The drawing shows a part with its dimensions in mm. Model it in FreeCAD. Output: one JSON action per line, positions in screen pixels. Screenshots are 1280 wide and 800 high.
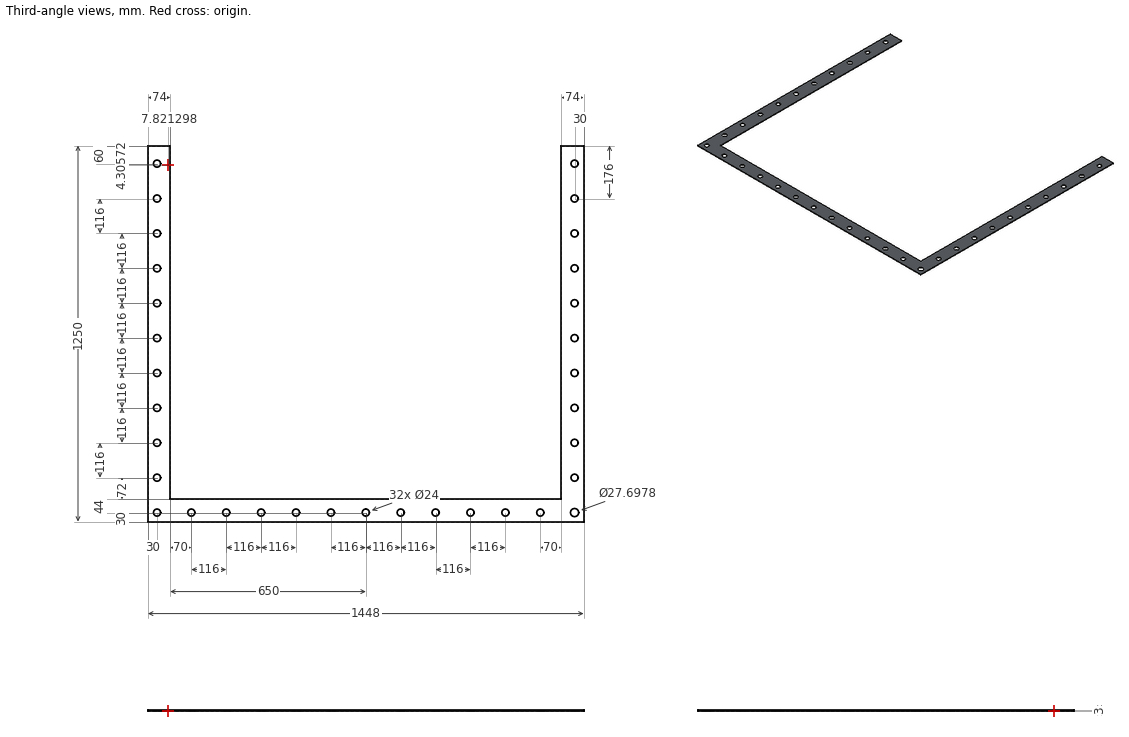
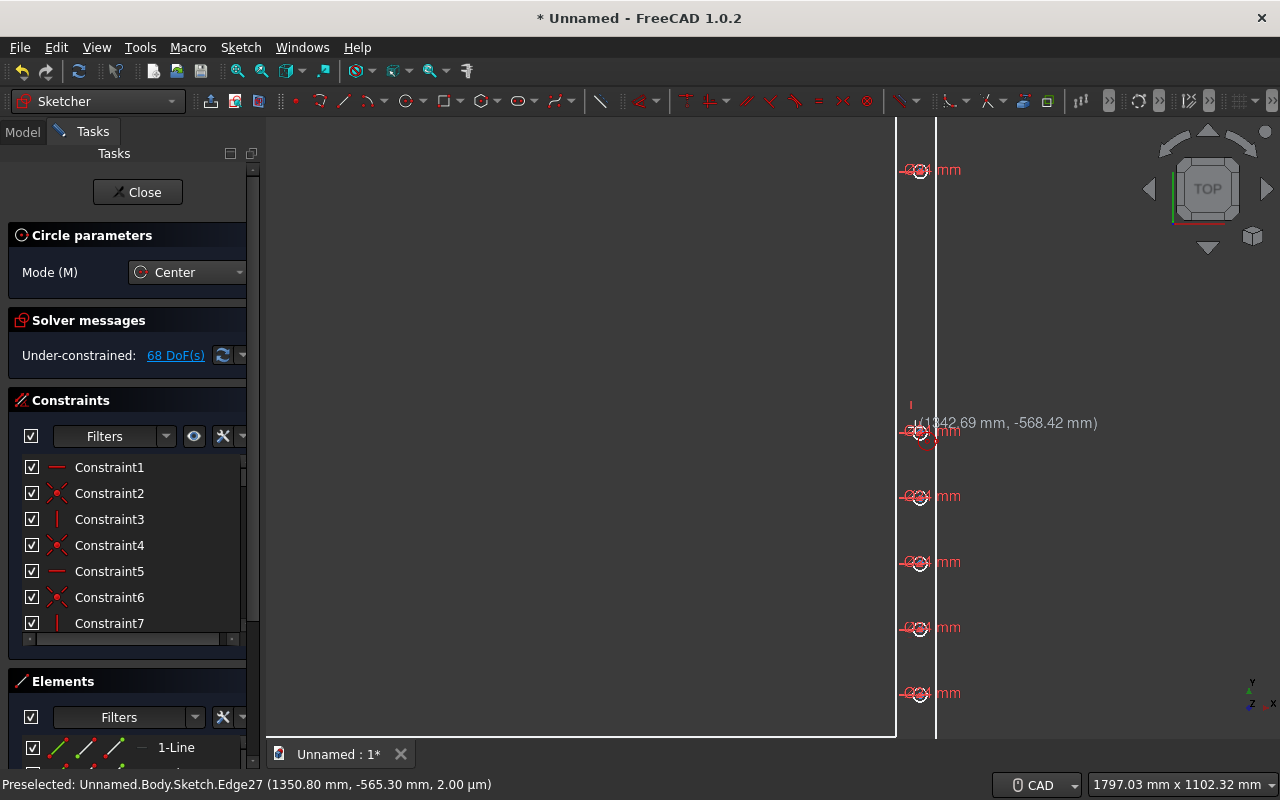
{"action": "scroll", "coordinate": [920, 367], "scroll_direction": "up", "scroll_amount": 7}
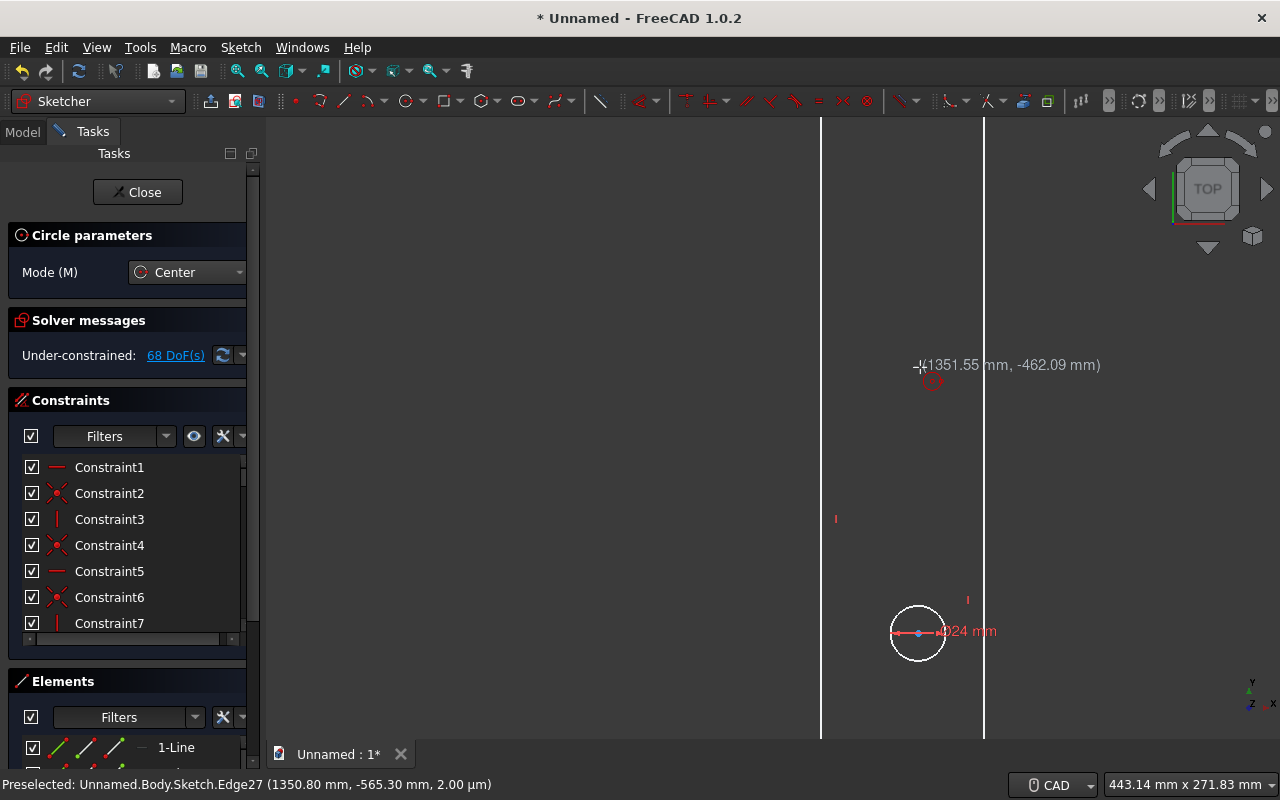
{"action": "scroll", "coordinate": [920, 402], "scroll_direction": "down", "scroll_amount": 10}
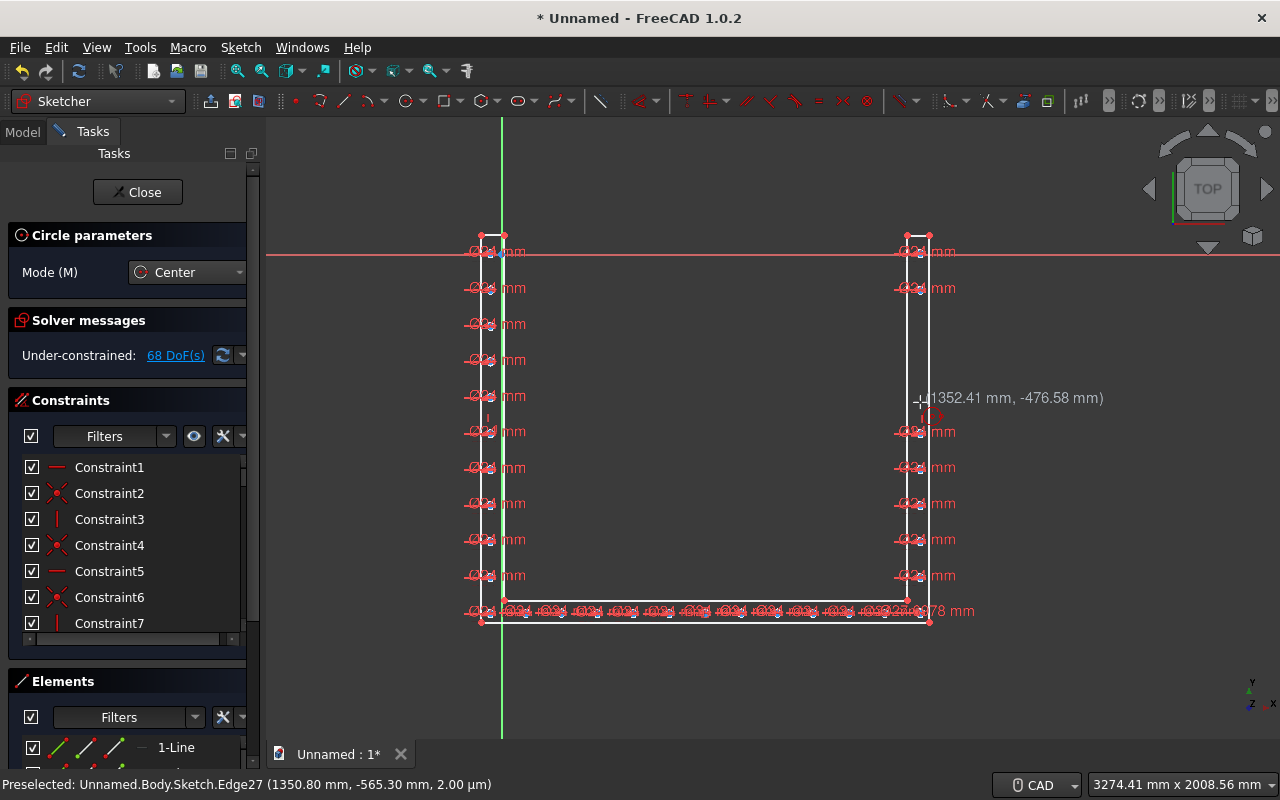
{"action": "scroll", "coordinate": [920, 397], "scroll_direction": "up", "scroll_amount": 3}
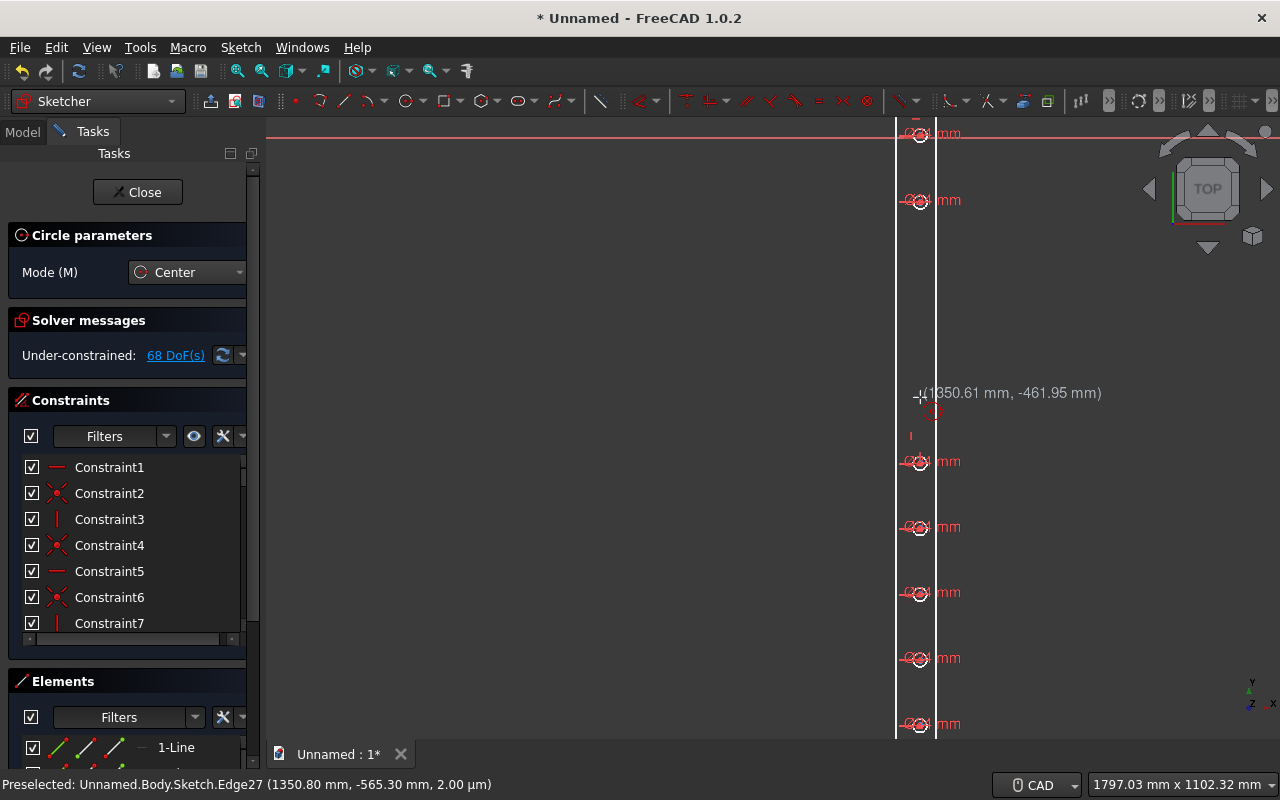
{"action": "left_click", "coordinate": [920, 397]}
{"action": "mouse_move", "coordinate": [915, 392]}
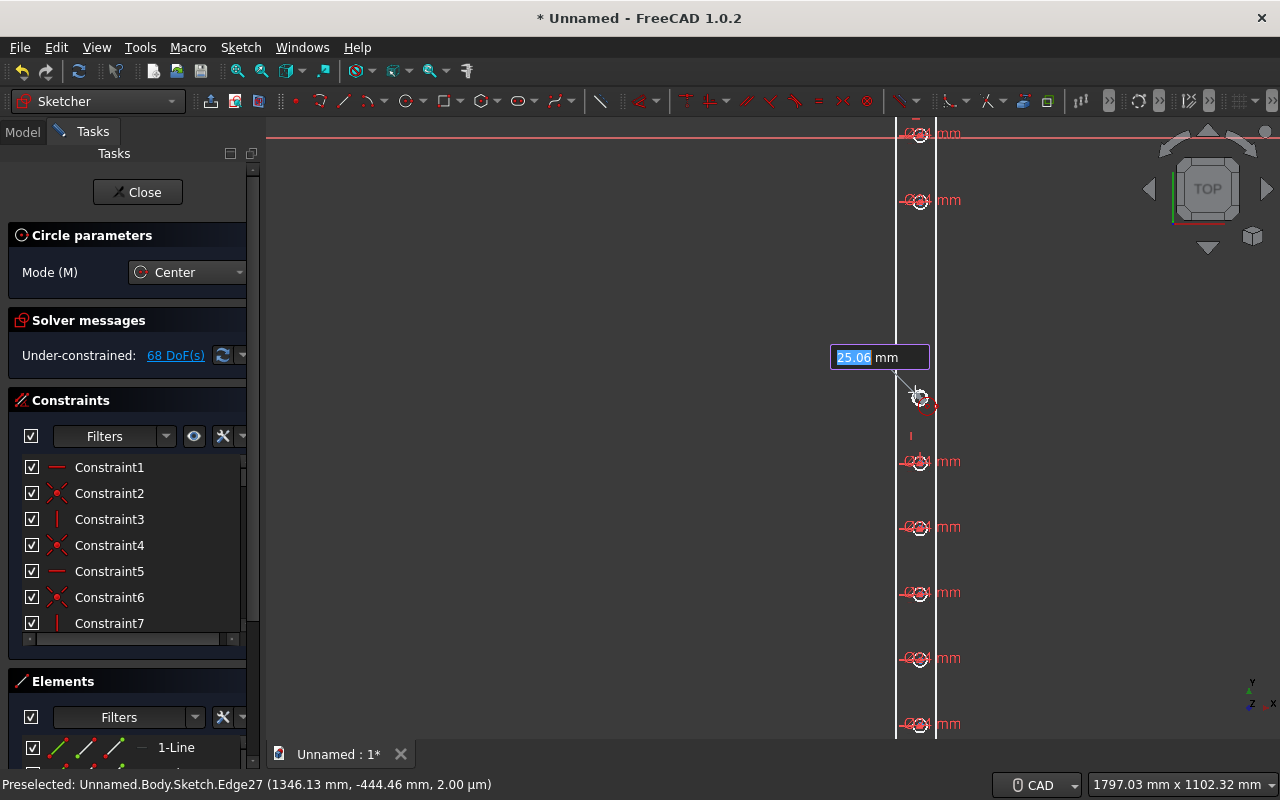
{"action": "type", "text": "24"}
{"action": "key", "text": "Return"}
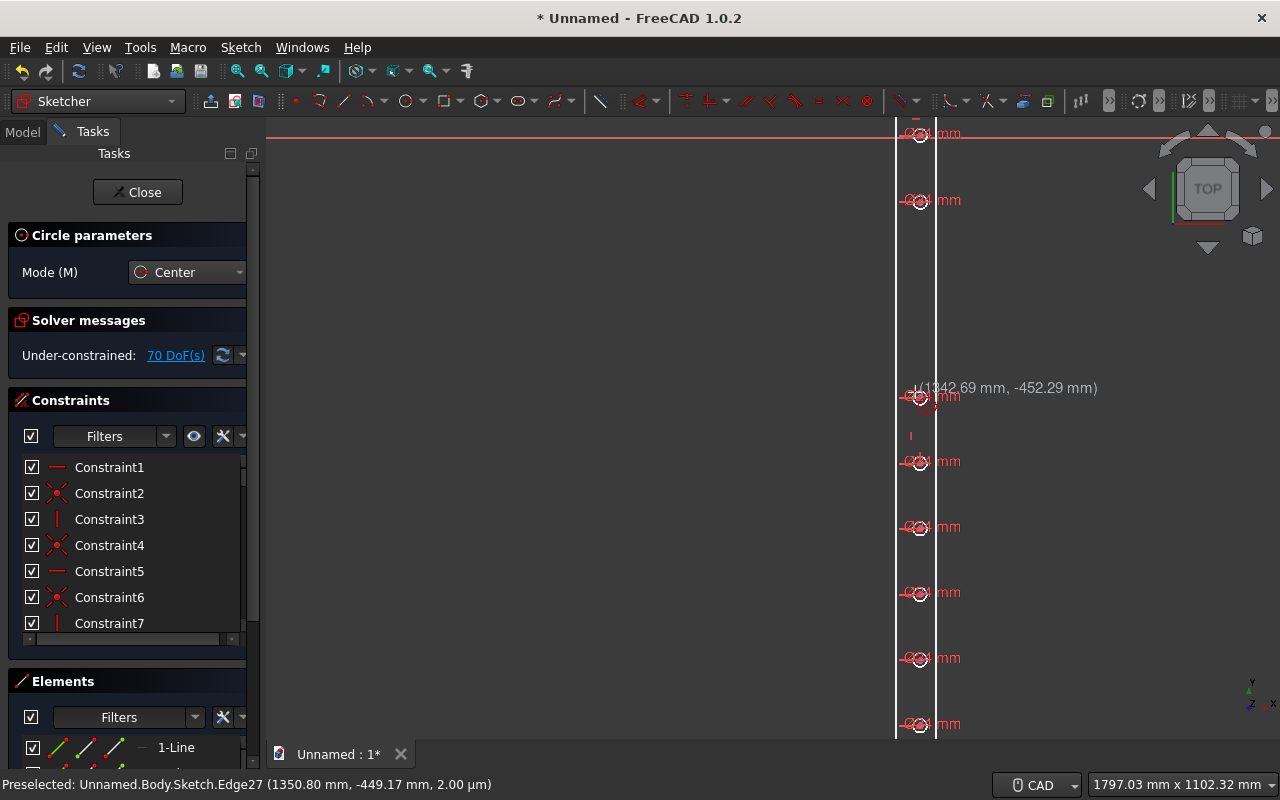
{"action": "scroll", "coordinate": [920, 332], "scroll_direction": "up", "scroll_amount": 7}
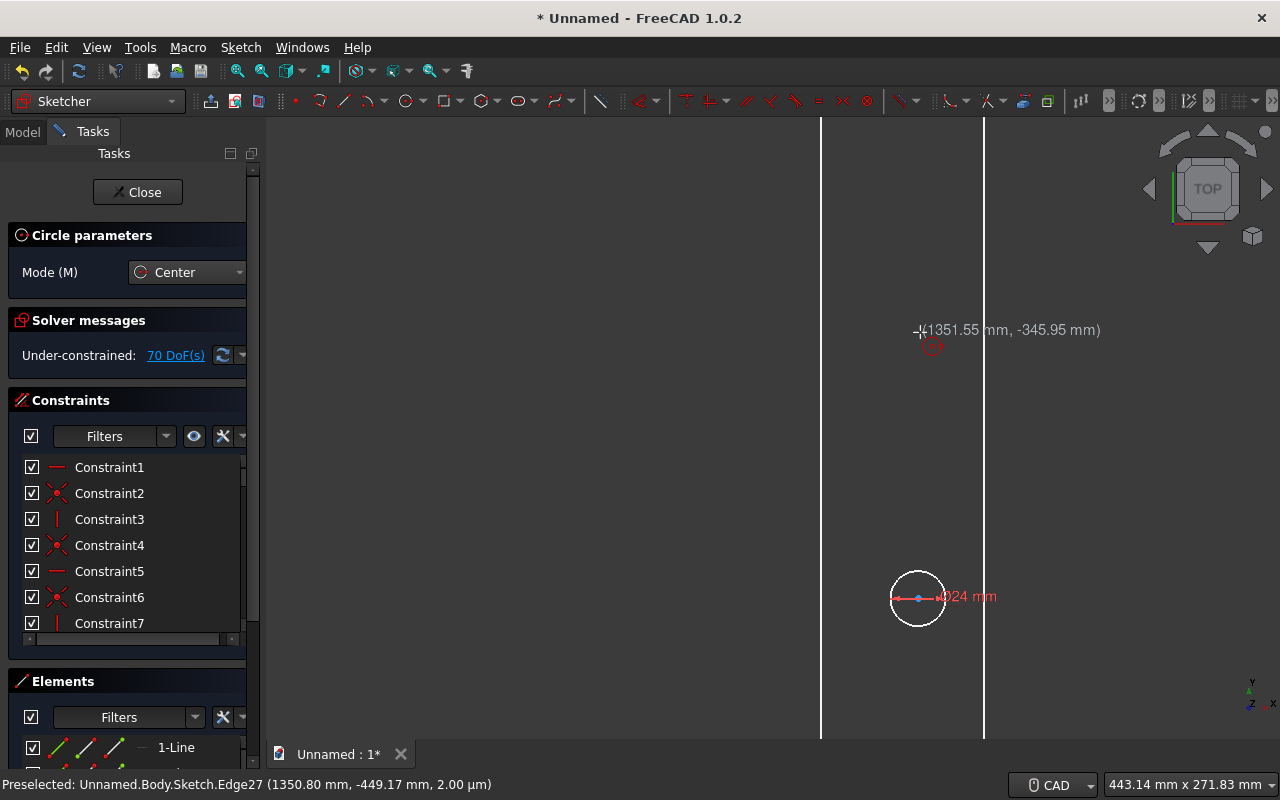
{"action": "scroll", "coordinate": [920, 366], "scroll_direction": "down", "scroll_amount": 10}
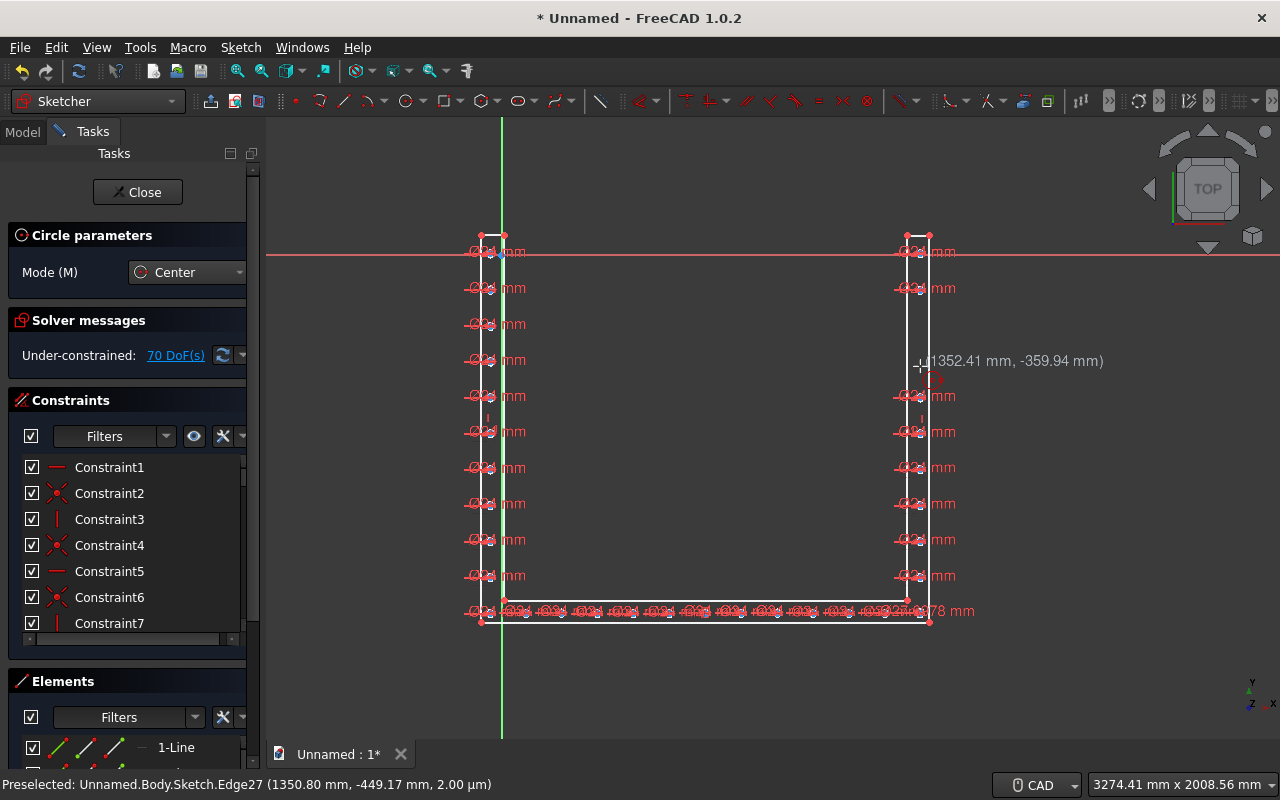
{"action": "scroll", "coordinate": [920, 361], "scroll_direction": "up", "scroll_amount": 3}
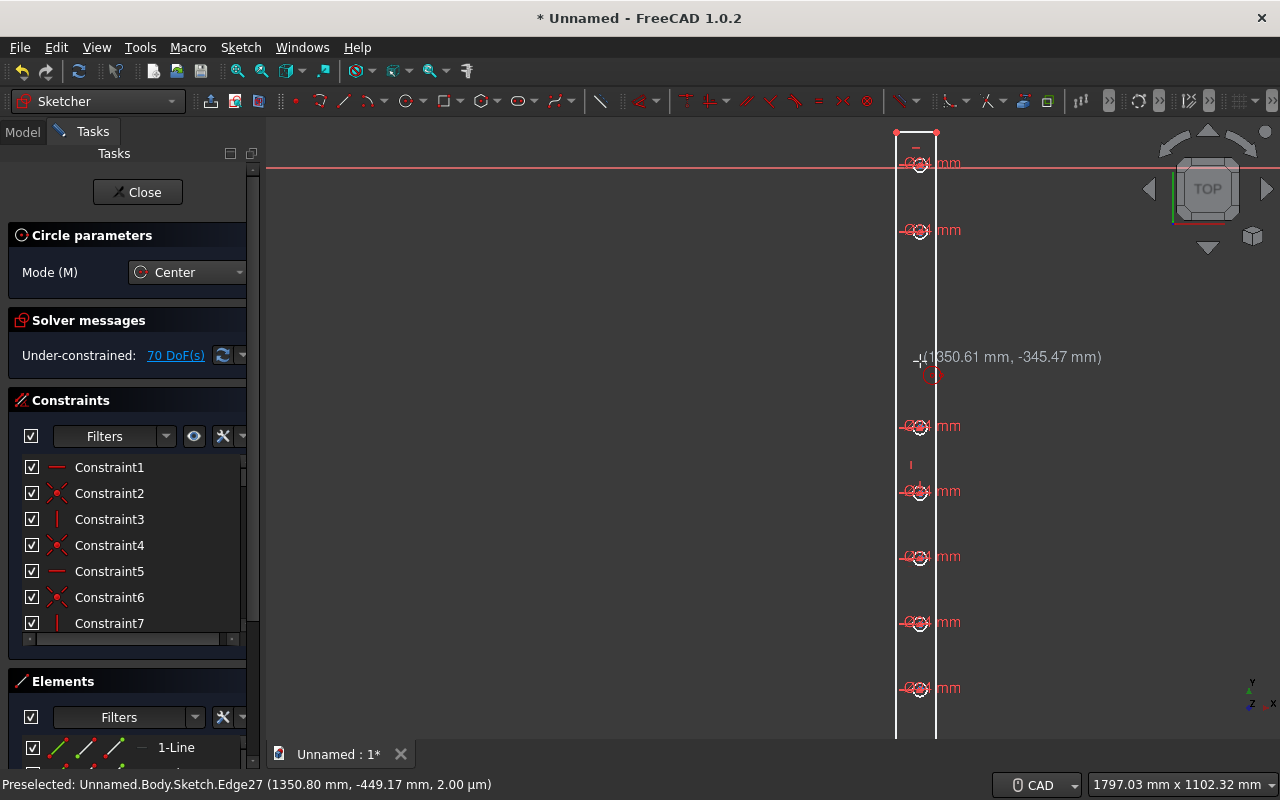
{"action": "left_click", "coordinate": [920, 361]}
{"action": "mouse_move", "coordinate": [915, 357]}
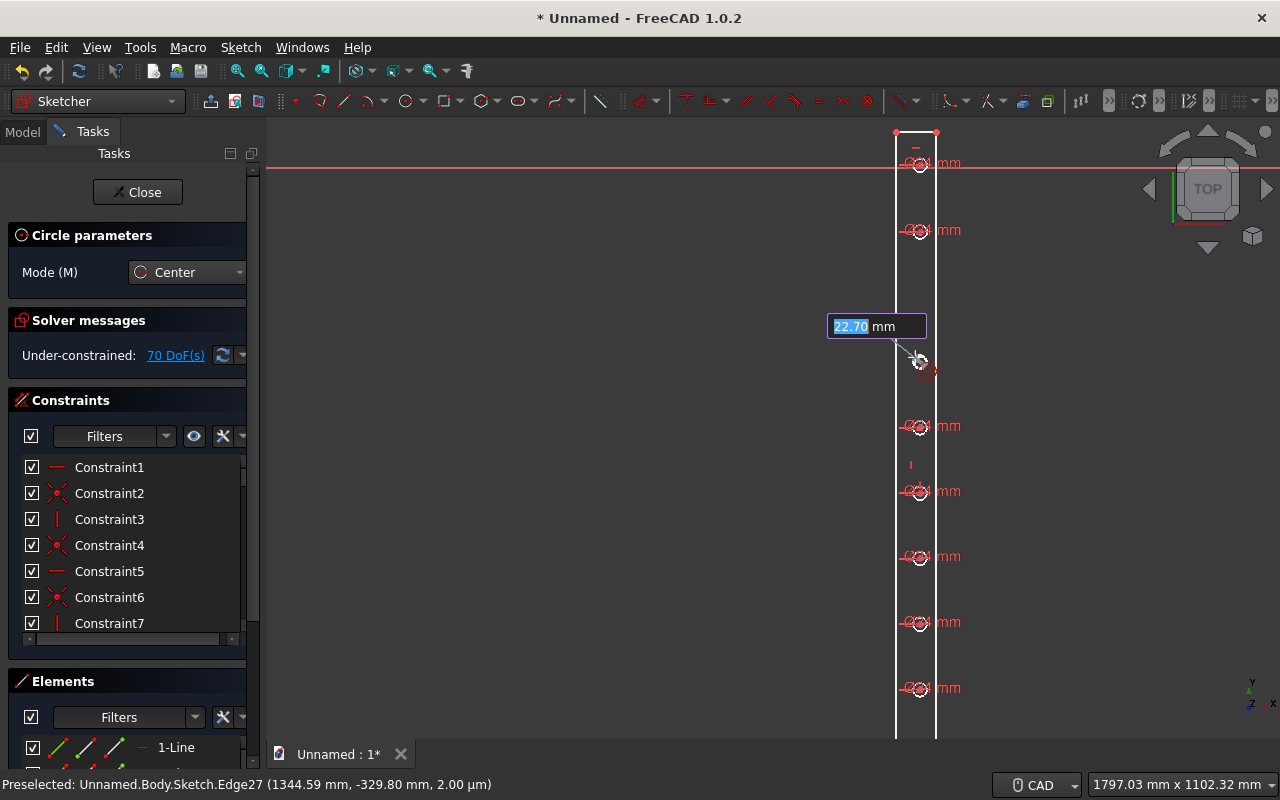
{"action": "type", "text": "24"}
{"action": "key", "text": "Return"}